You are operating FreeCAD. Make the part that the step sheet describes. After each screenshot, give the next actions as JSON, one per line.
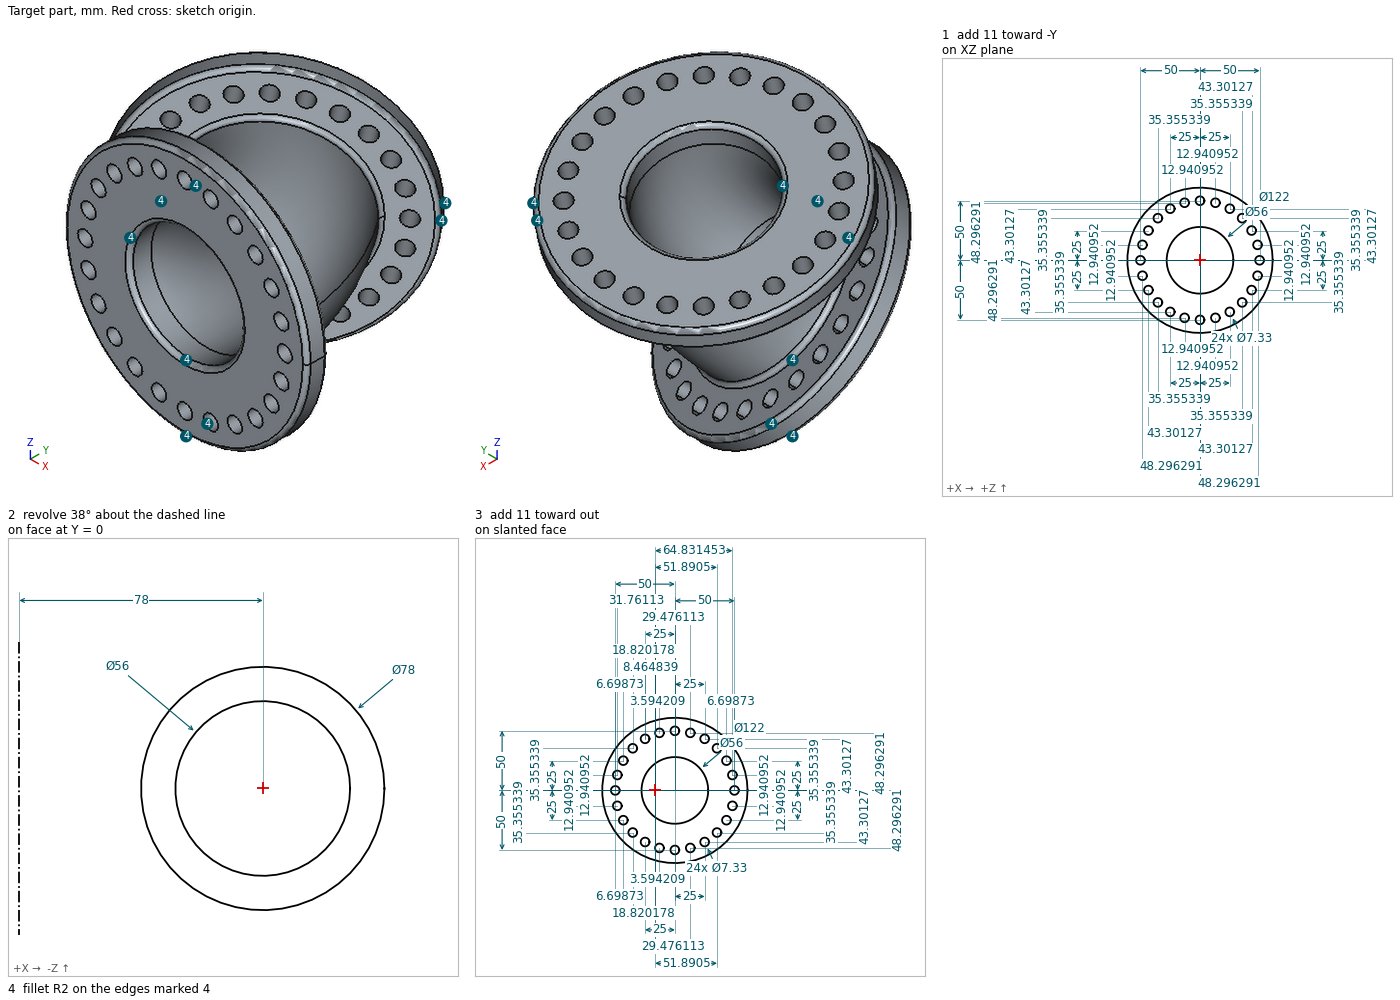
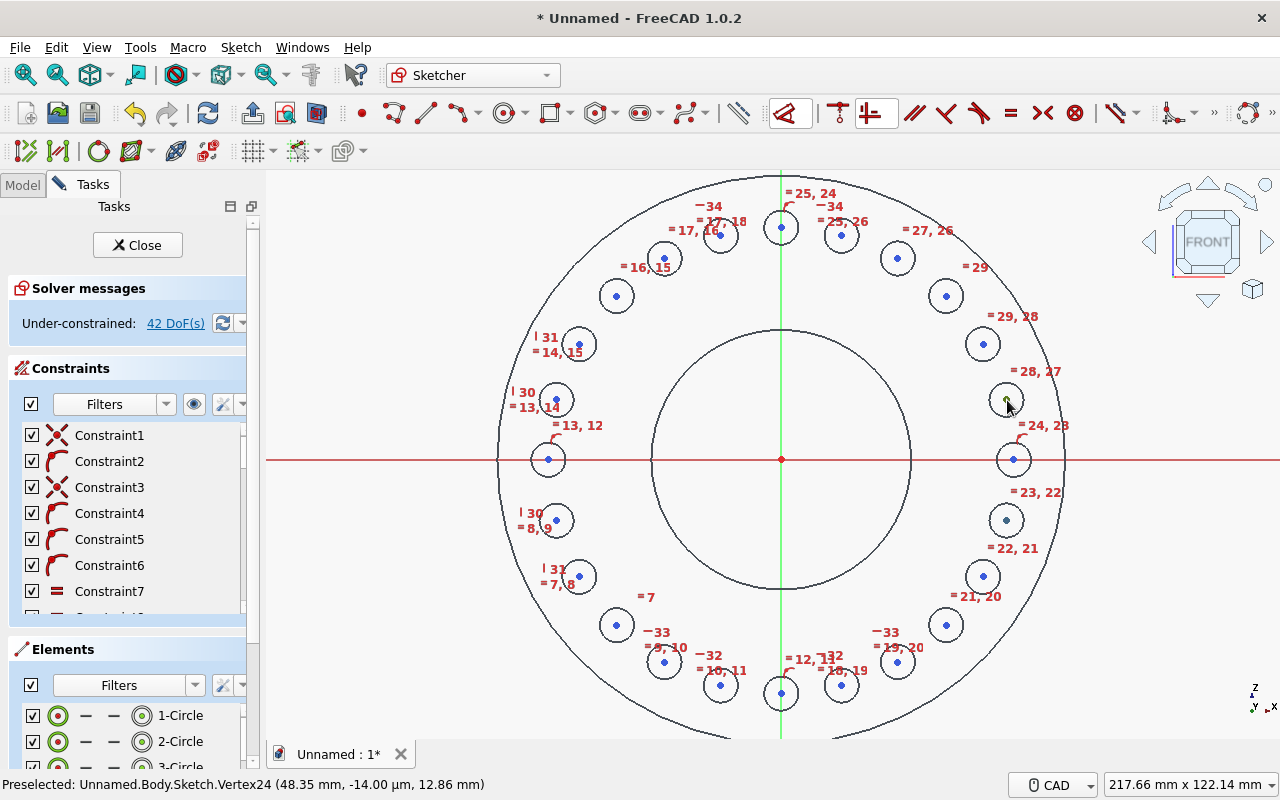
{"action": "key", "text": "v"}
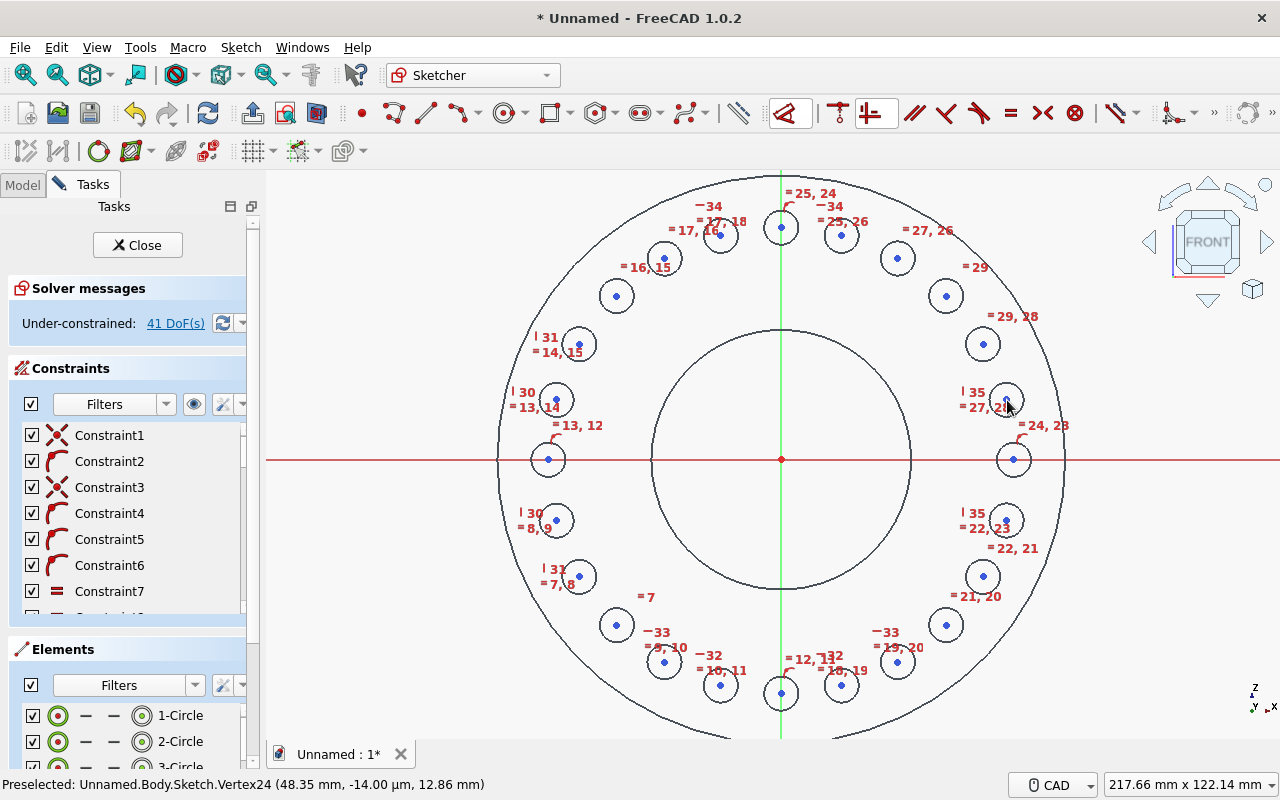
{"action": "left_click", "coordinate": [784, 114]}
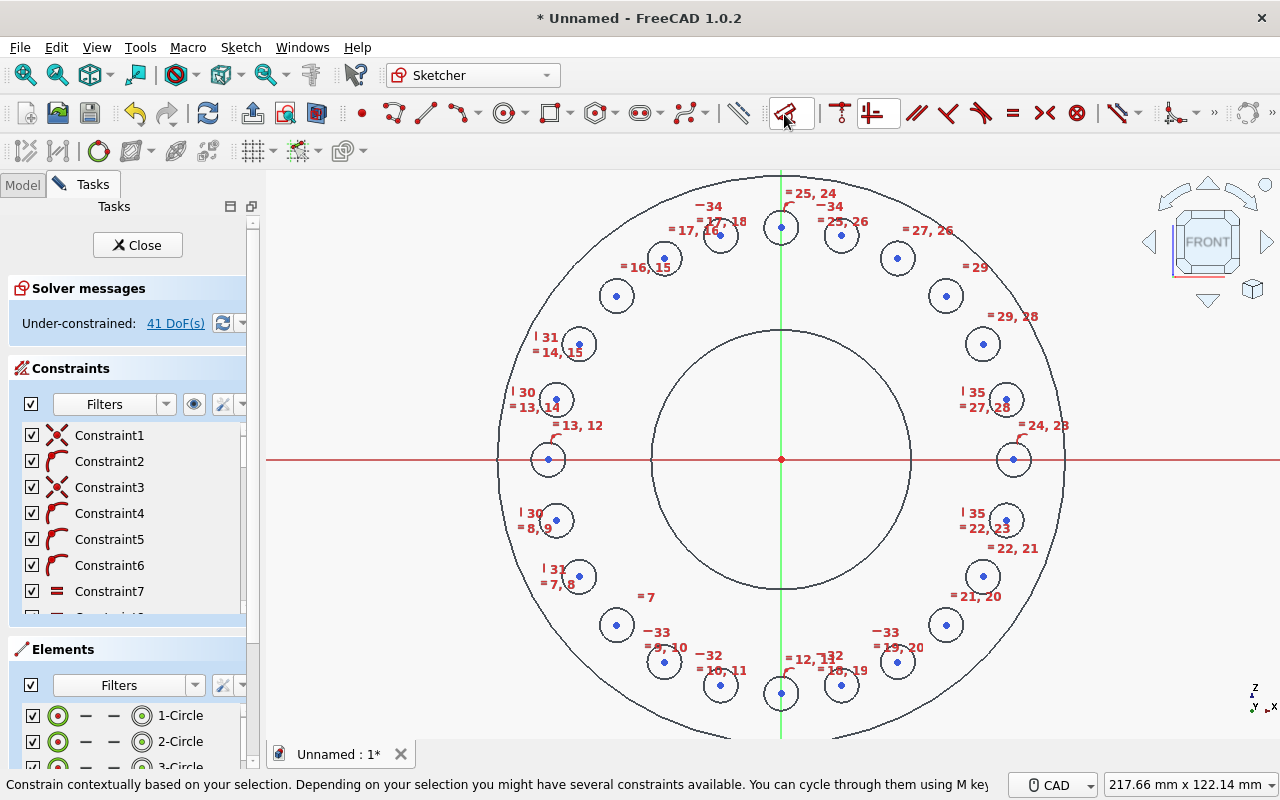
{"action": "left_click", "coordinate": [981, 258]}
{"action": "left_click", "coordinate": [1004, 235]}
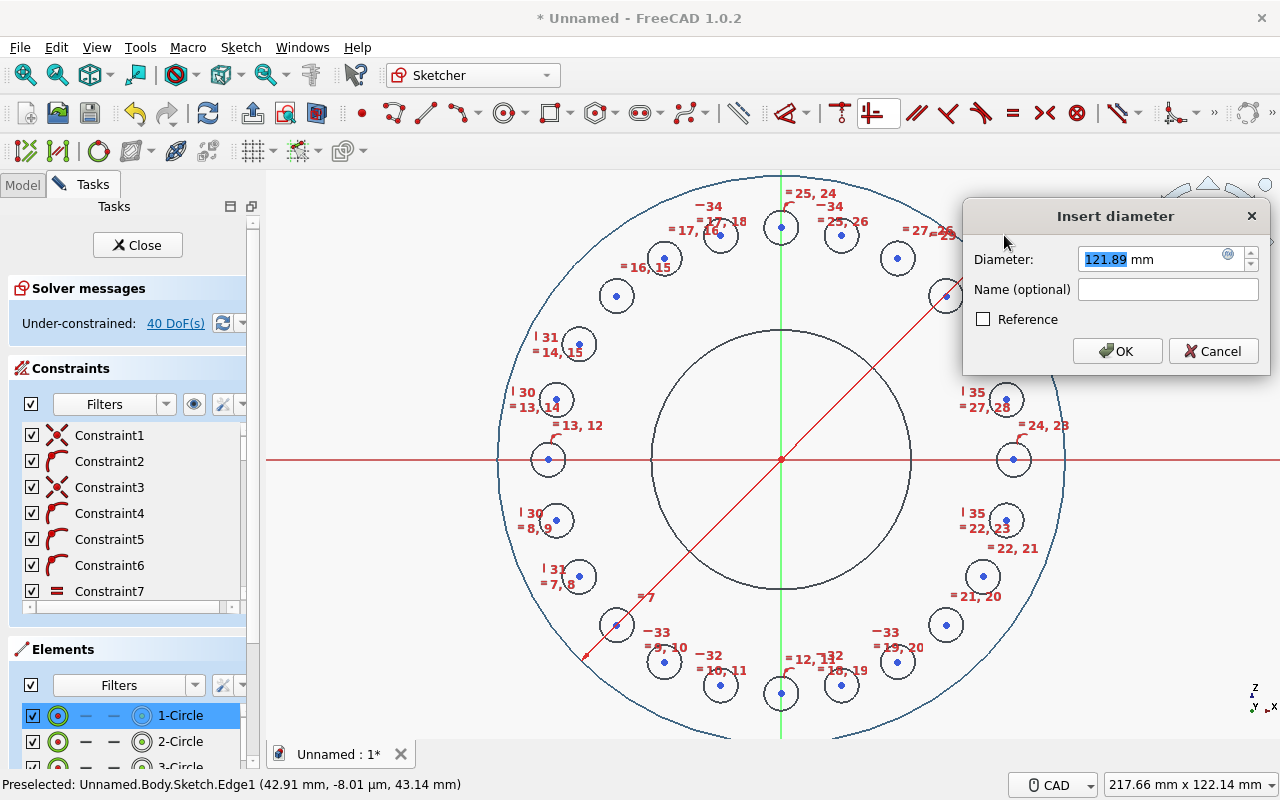
{"action": "type", "text": "122"}
{"action": "key", "text": "Return"}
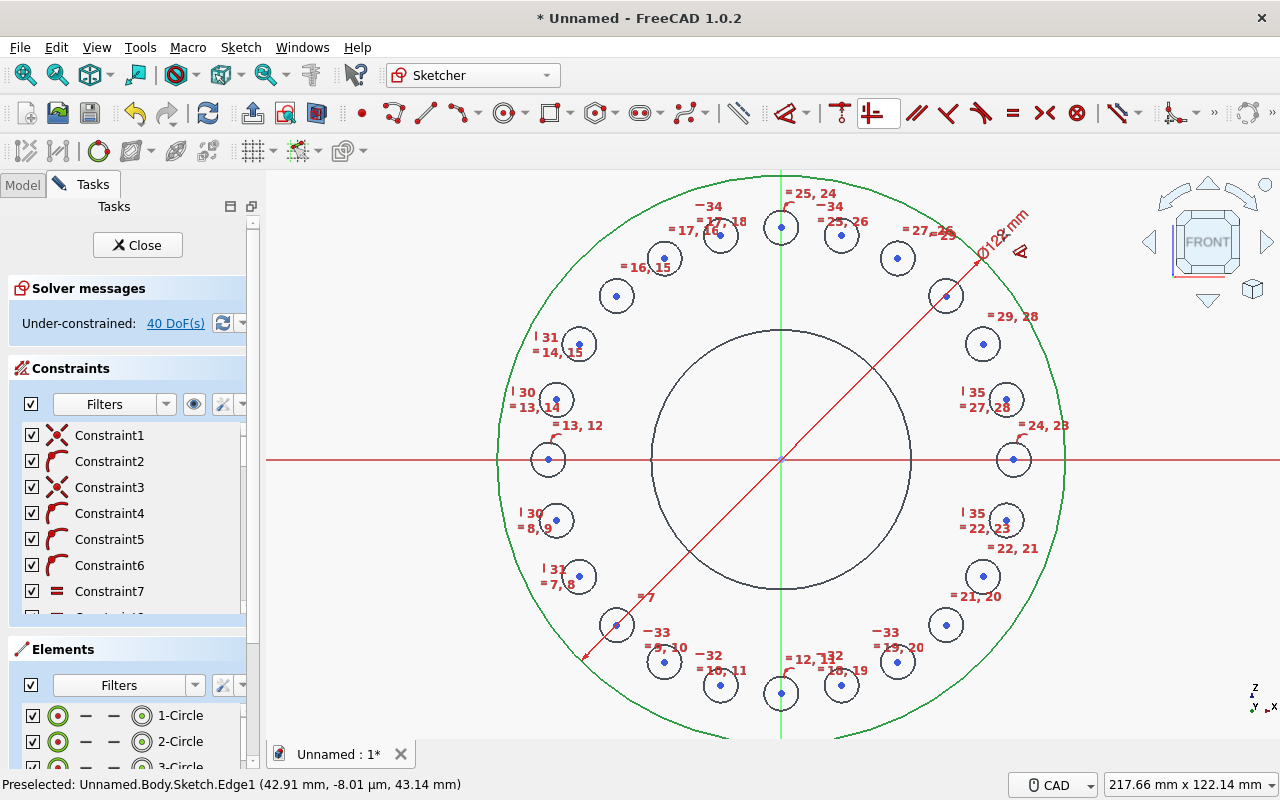
{"action": "left_click", "coordinate": [629, 613]}
{"action": "left_click", "coordinate": [652, 590]}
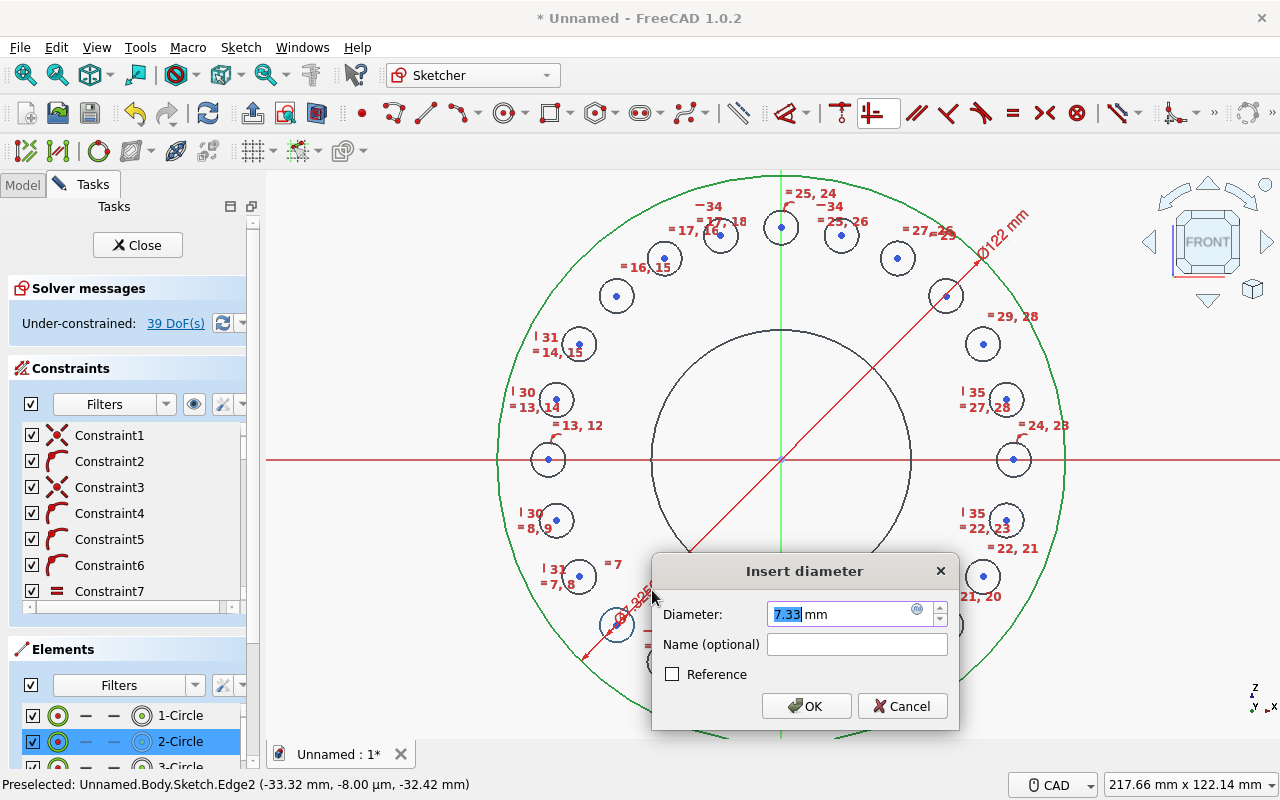
{"action": "type", "text": "7.33"}
{"action": "key", "text": "Return"}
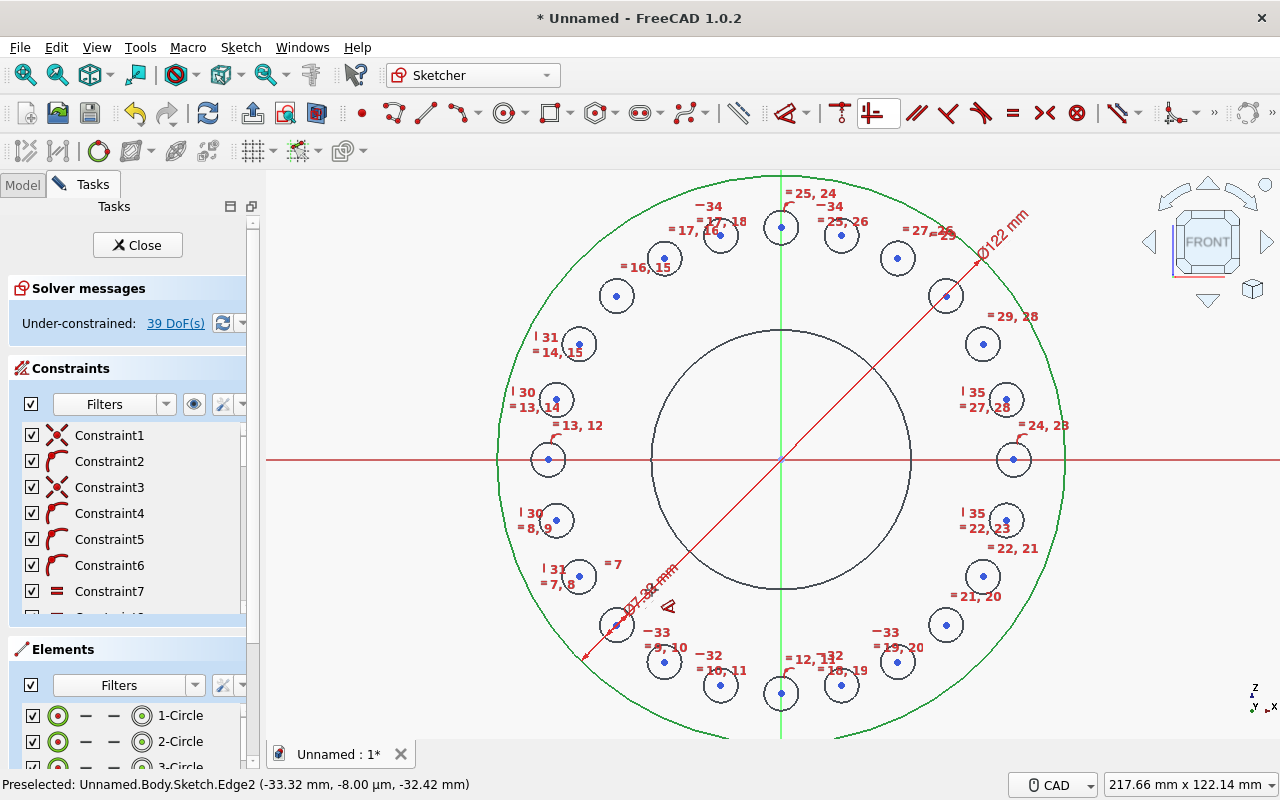
{"action": "left_click", "coordinate": [873, 368]}
{"action": "left_click", "coordinate": [896, 345]}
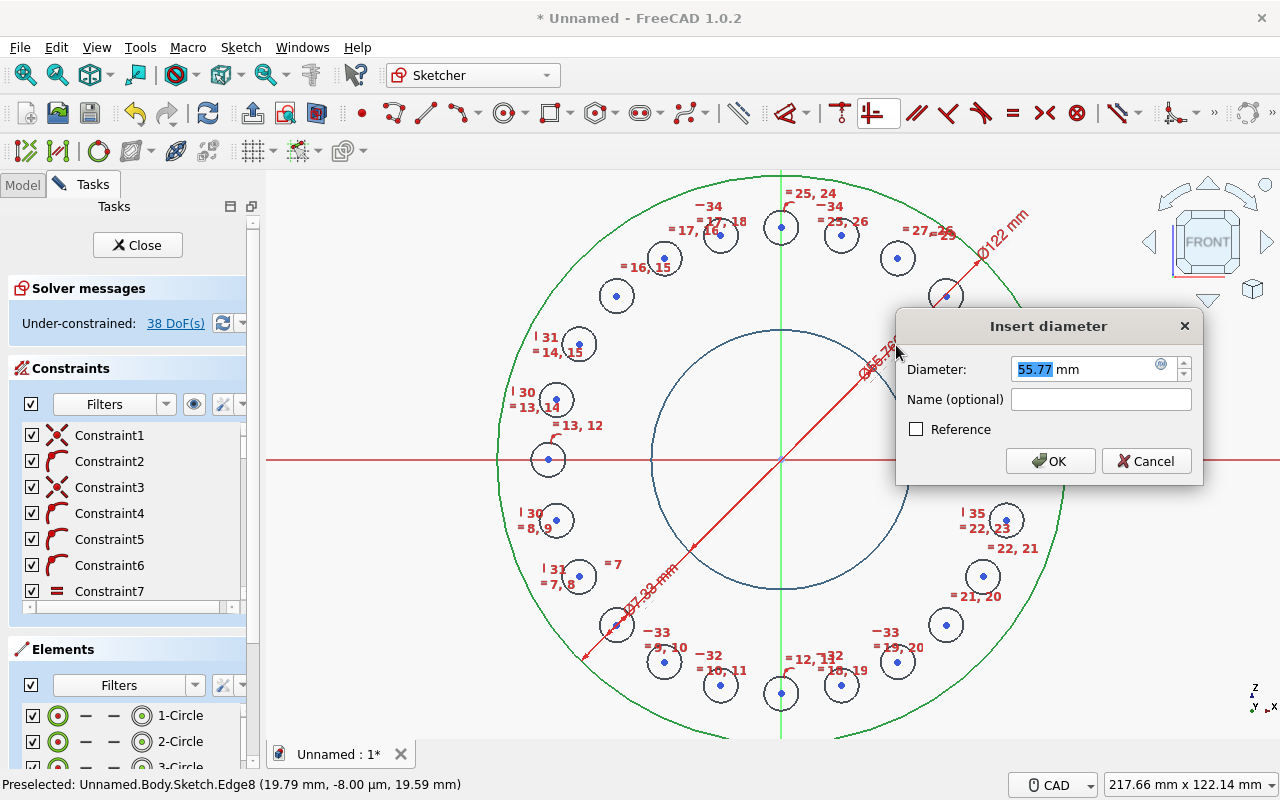
{"action": "type", "text": "56"}
{"action": "key", "text": "Return"}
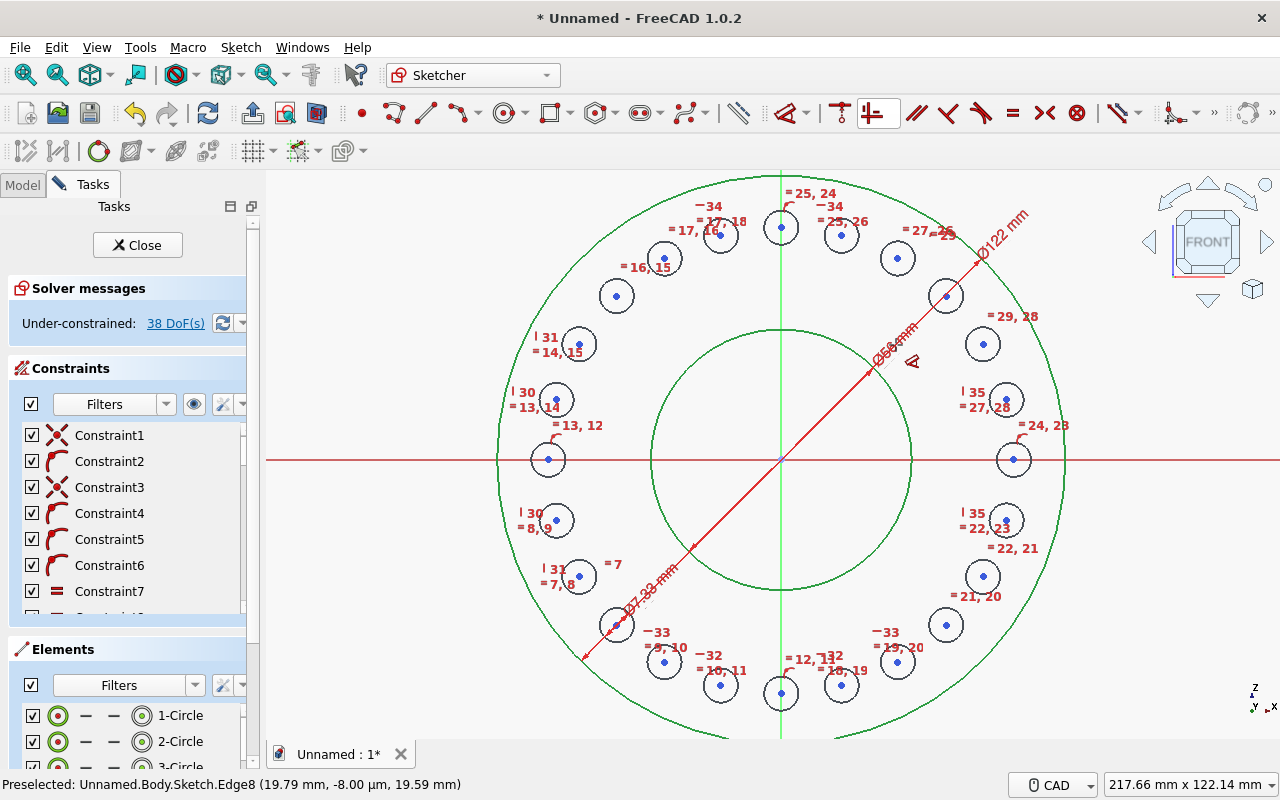
{"action": "left_click", "coordinate": [579, 577]}
{"action": "left_click", "coordinate": [545, 491]}